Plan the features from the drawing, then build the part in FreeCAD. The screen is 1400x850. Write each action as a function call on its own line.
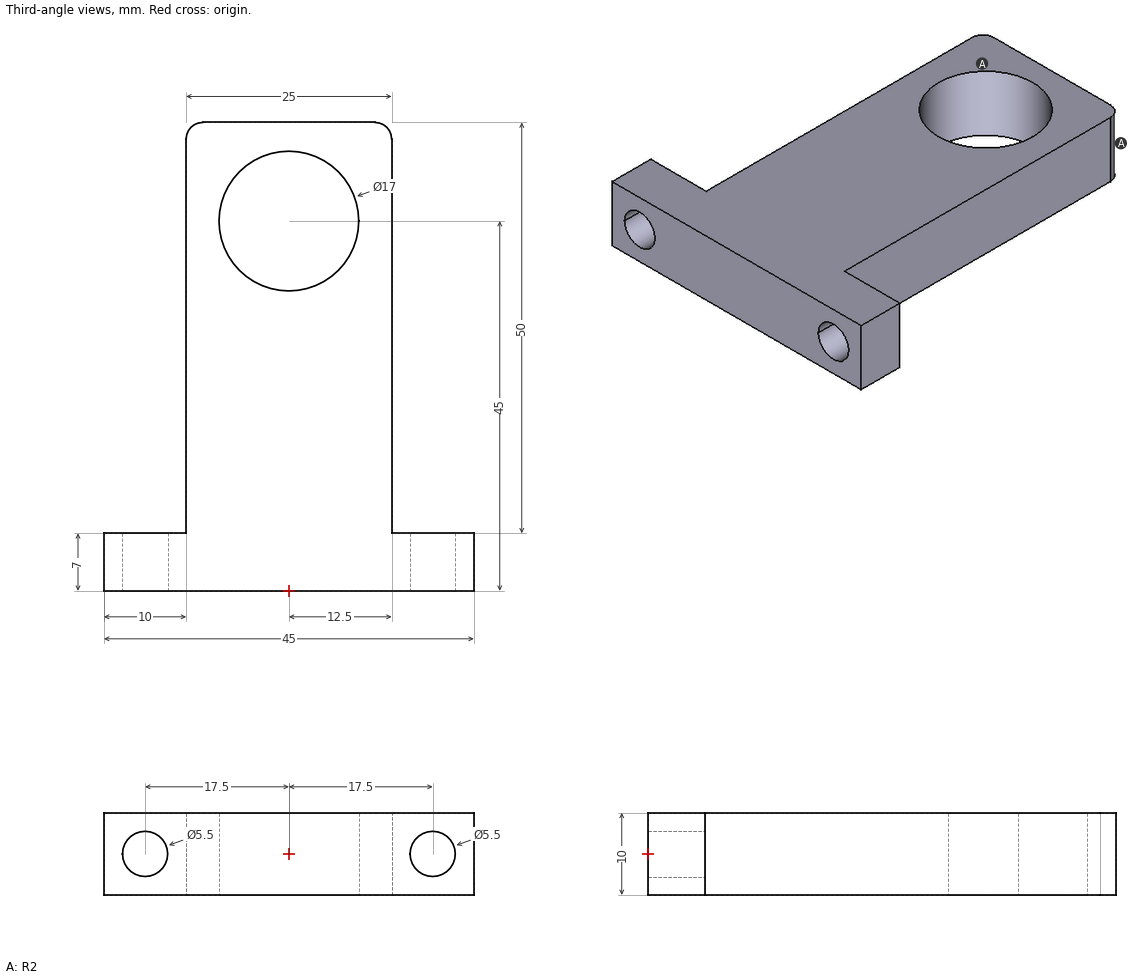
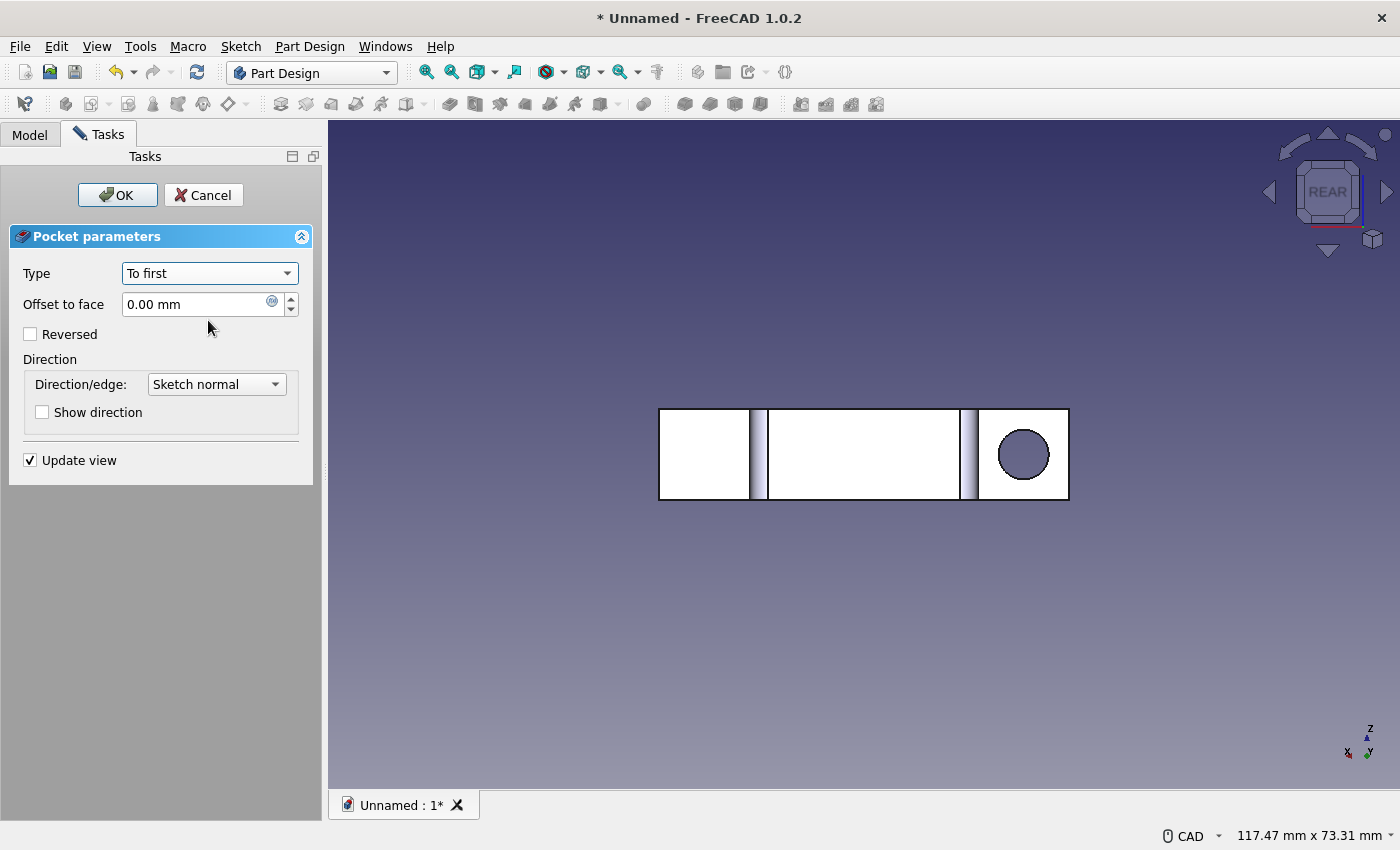
click(118, 195)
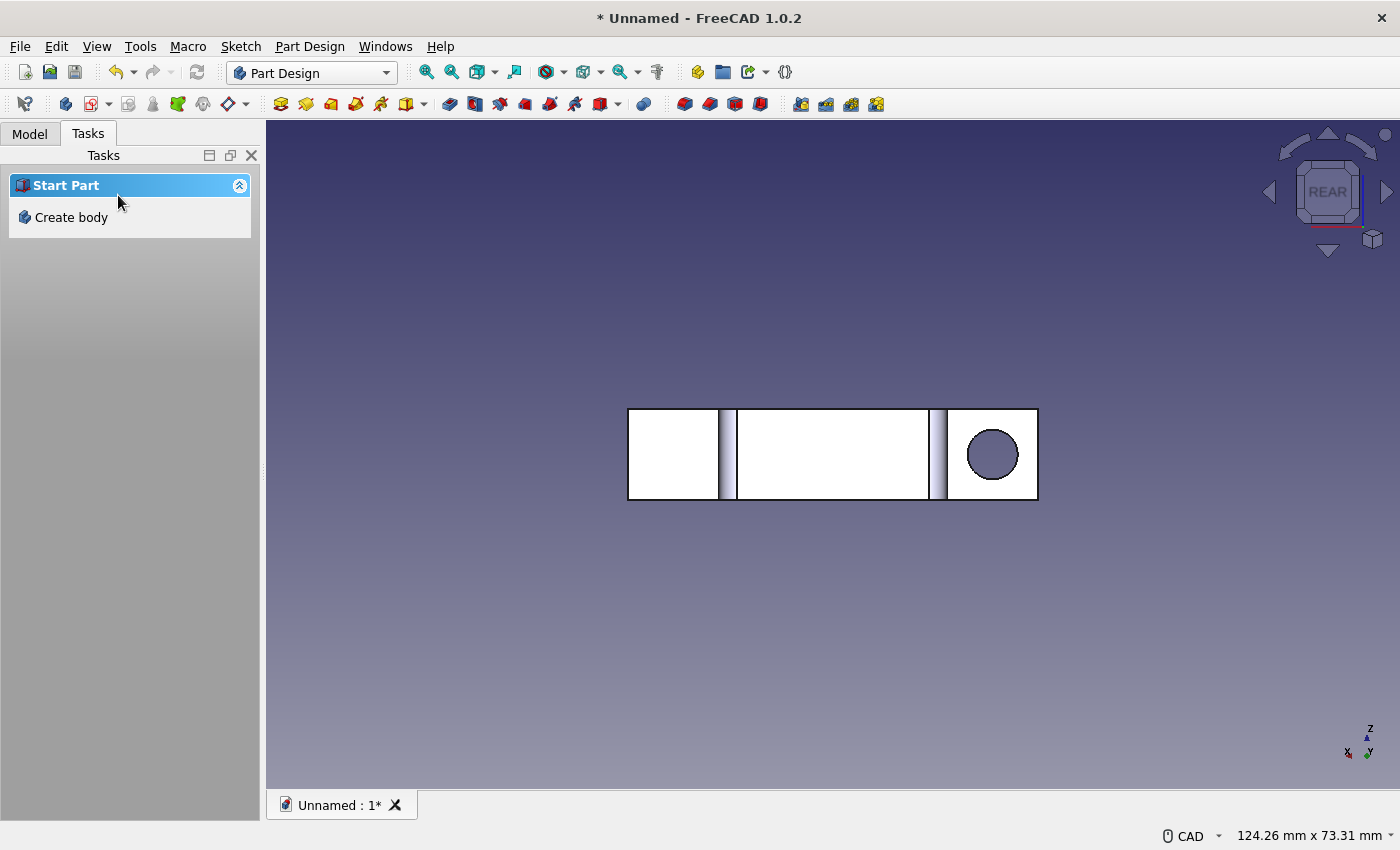
key(v)
key(f)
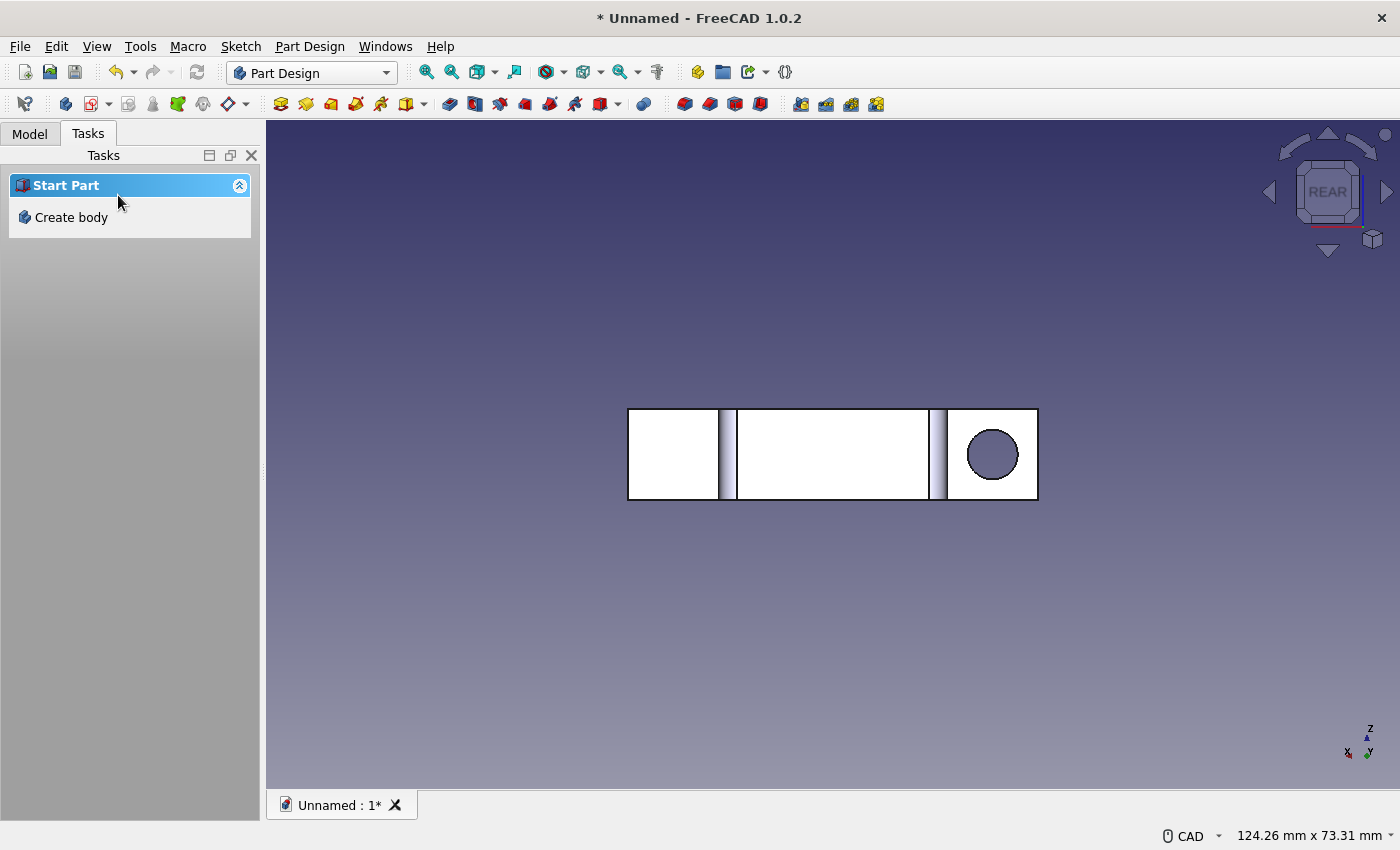
click(673, 453)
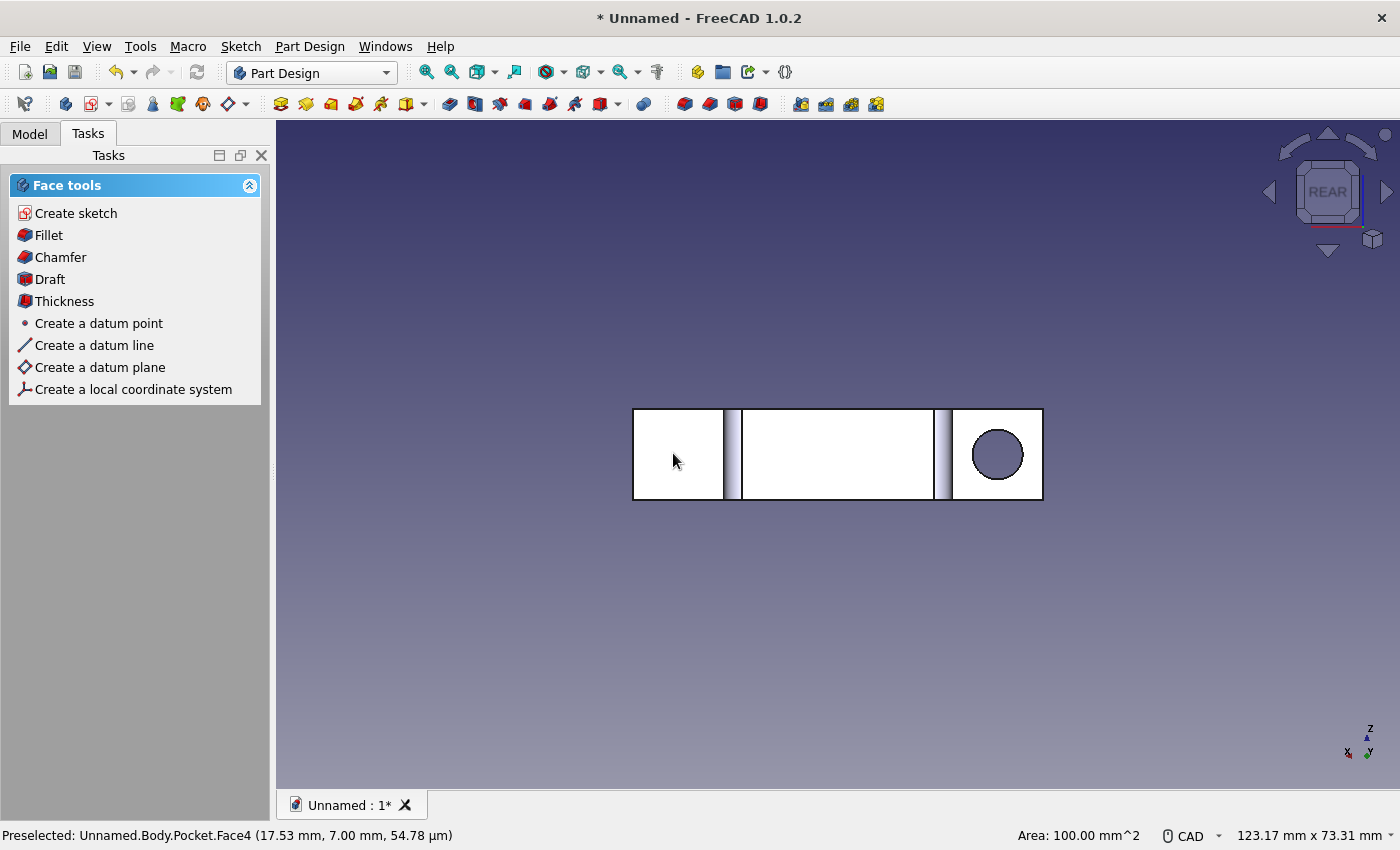
click(90, 104)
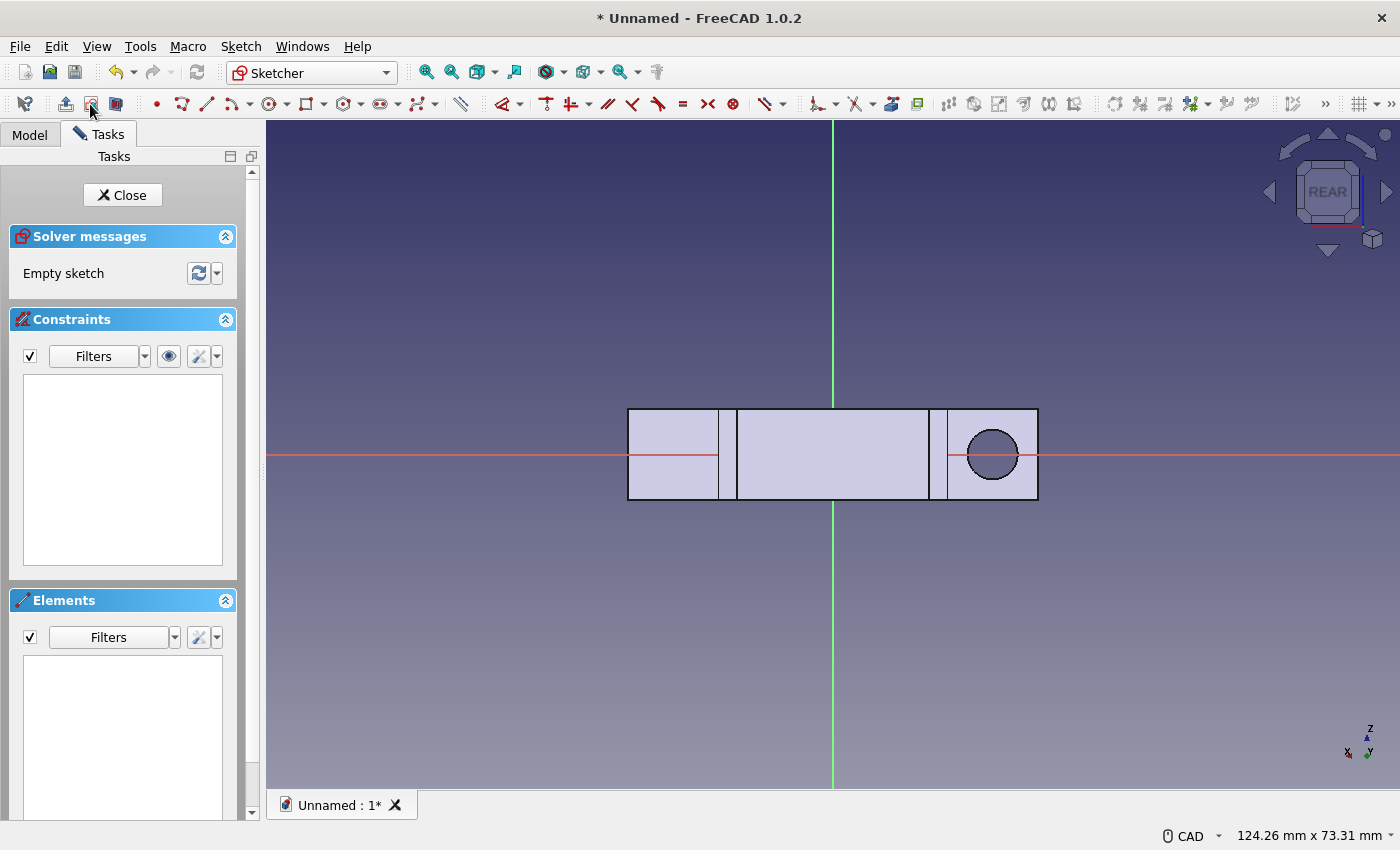
click(116, 104)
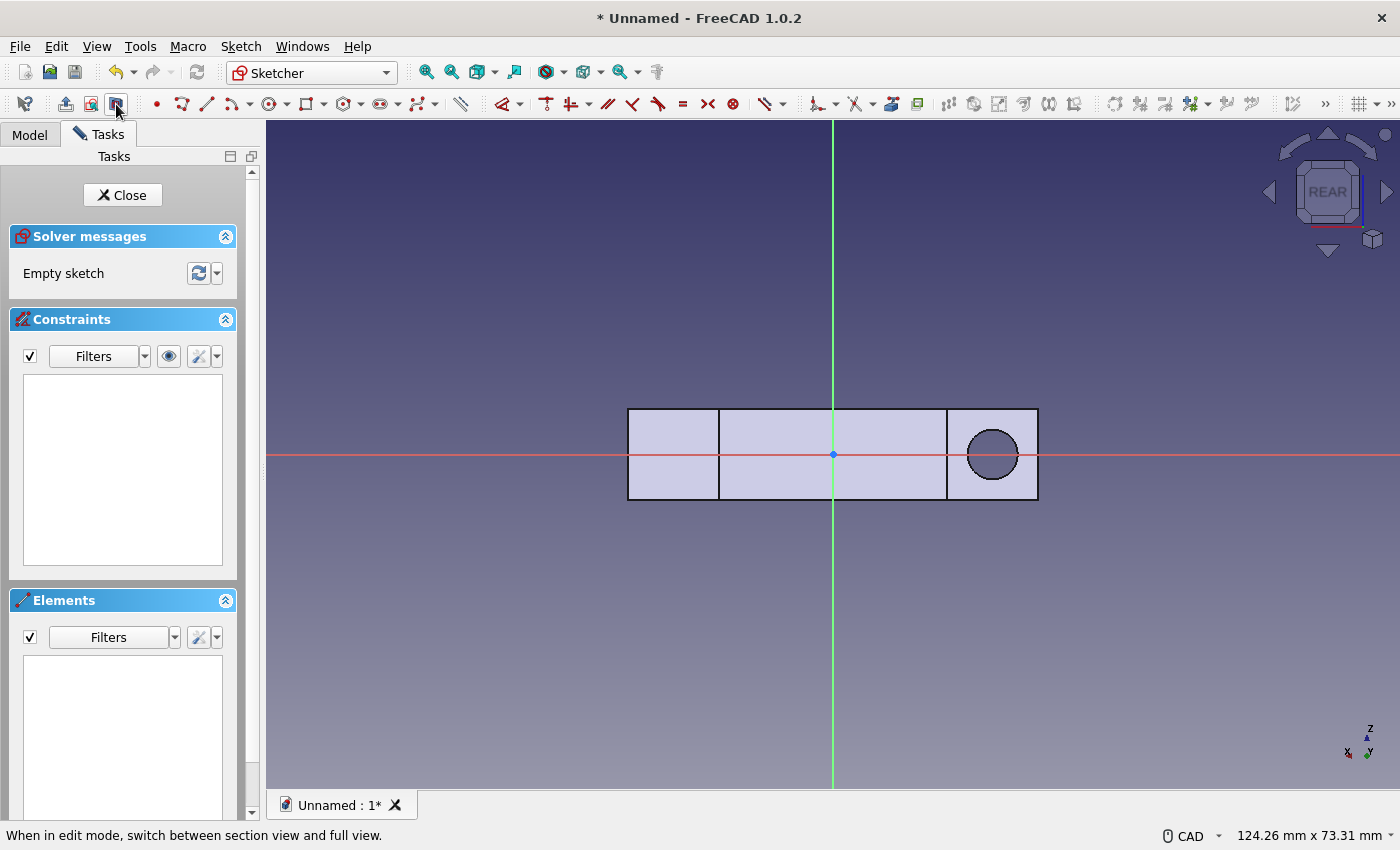
scroll(662, 454, up, 11)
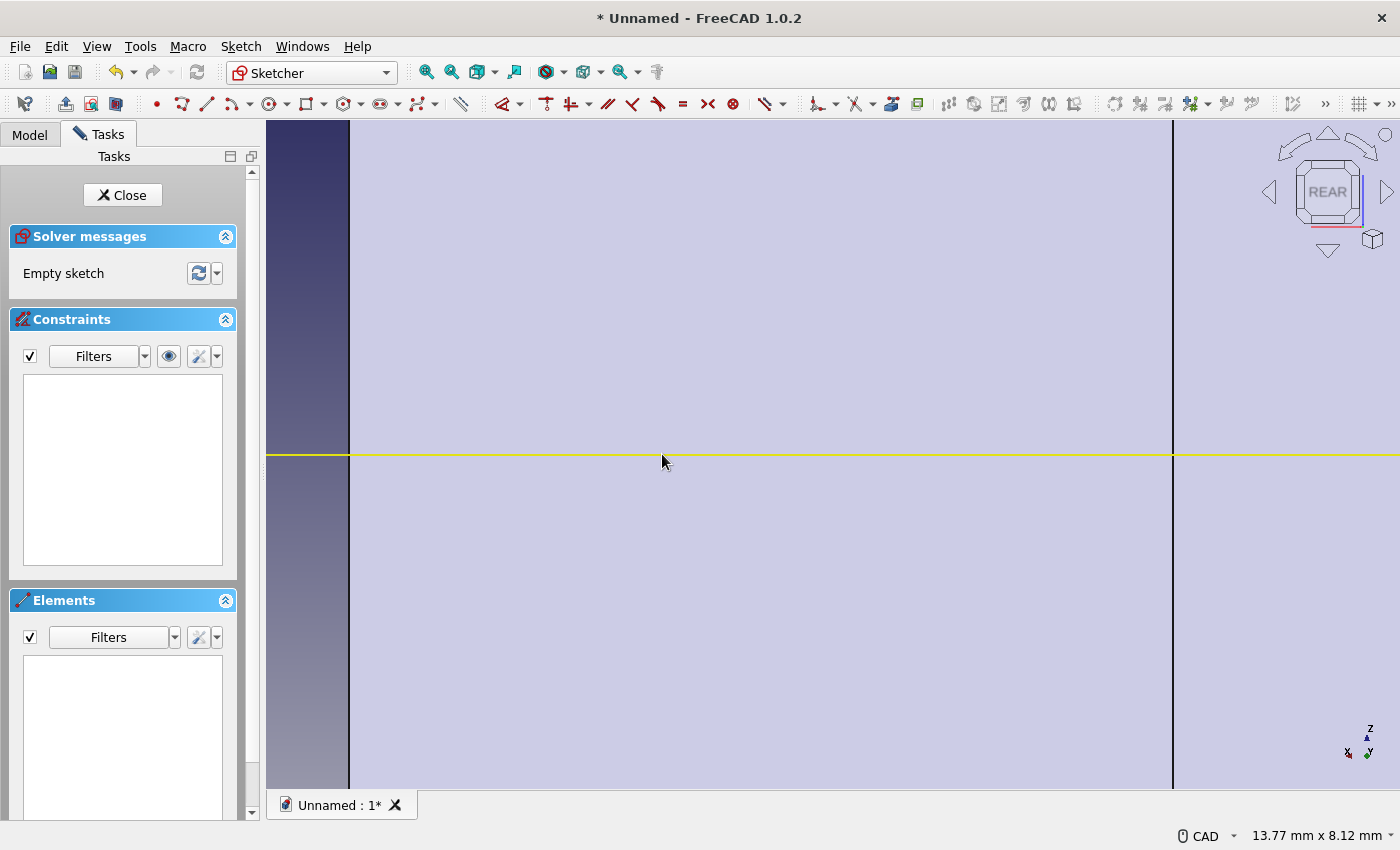
key(g)
key(c)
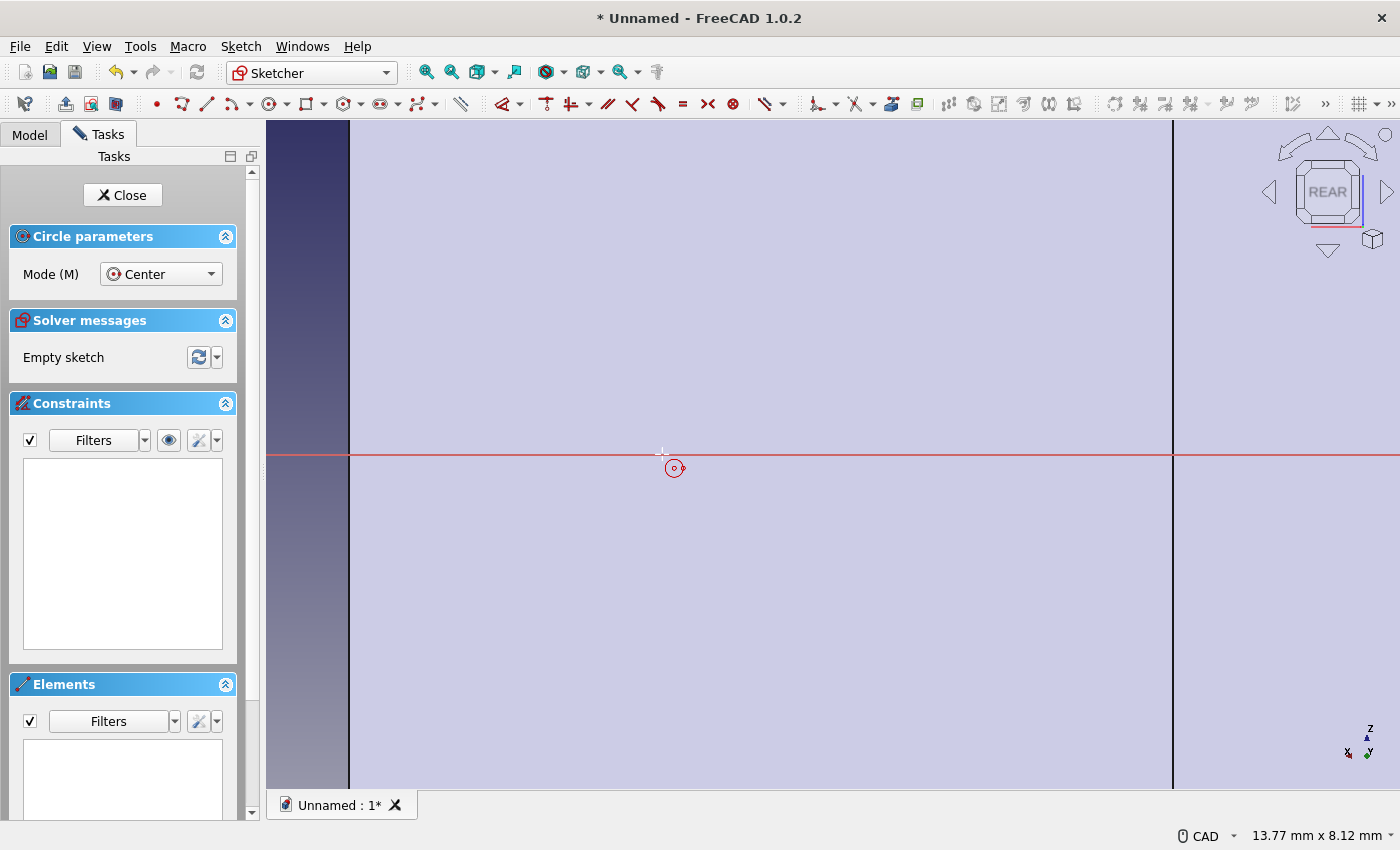
click(761, 454)
click(921, 294)
key(Escape)